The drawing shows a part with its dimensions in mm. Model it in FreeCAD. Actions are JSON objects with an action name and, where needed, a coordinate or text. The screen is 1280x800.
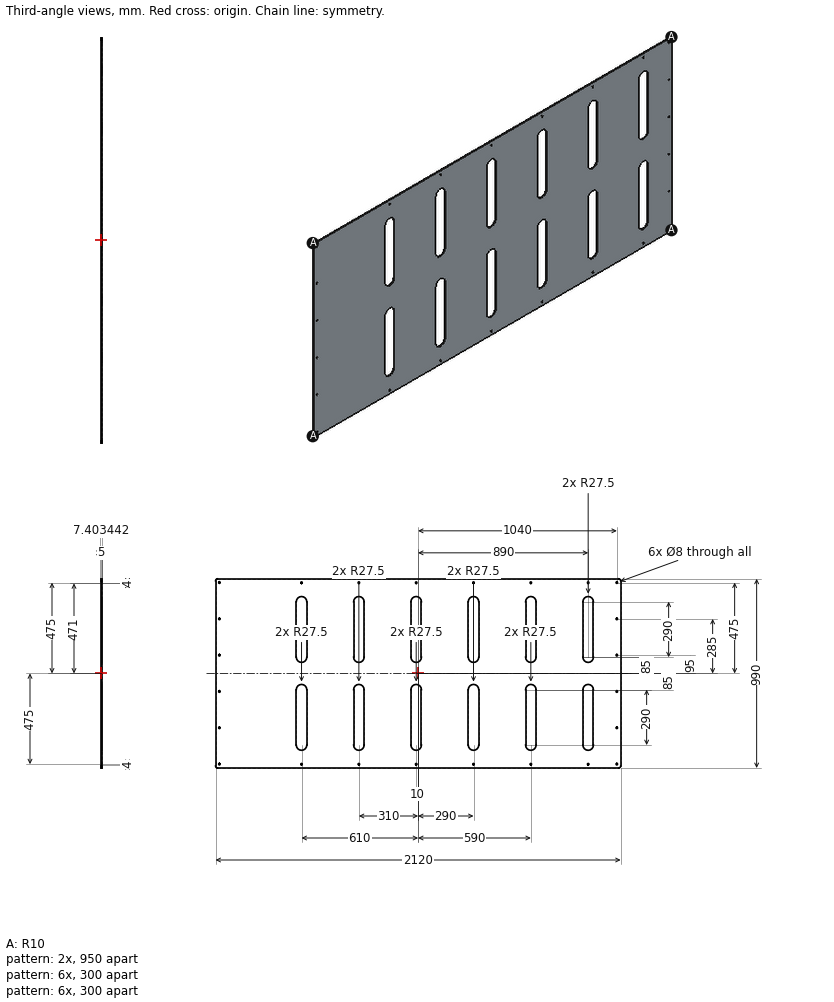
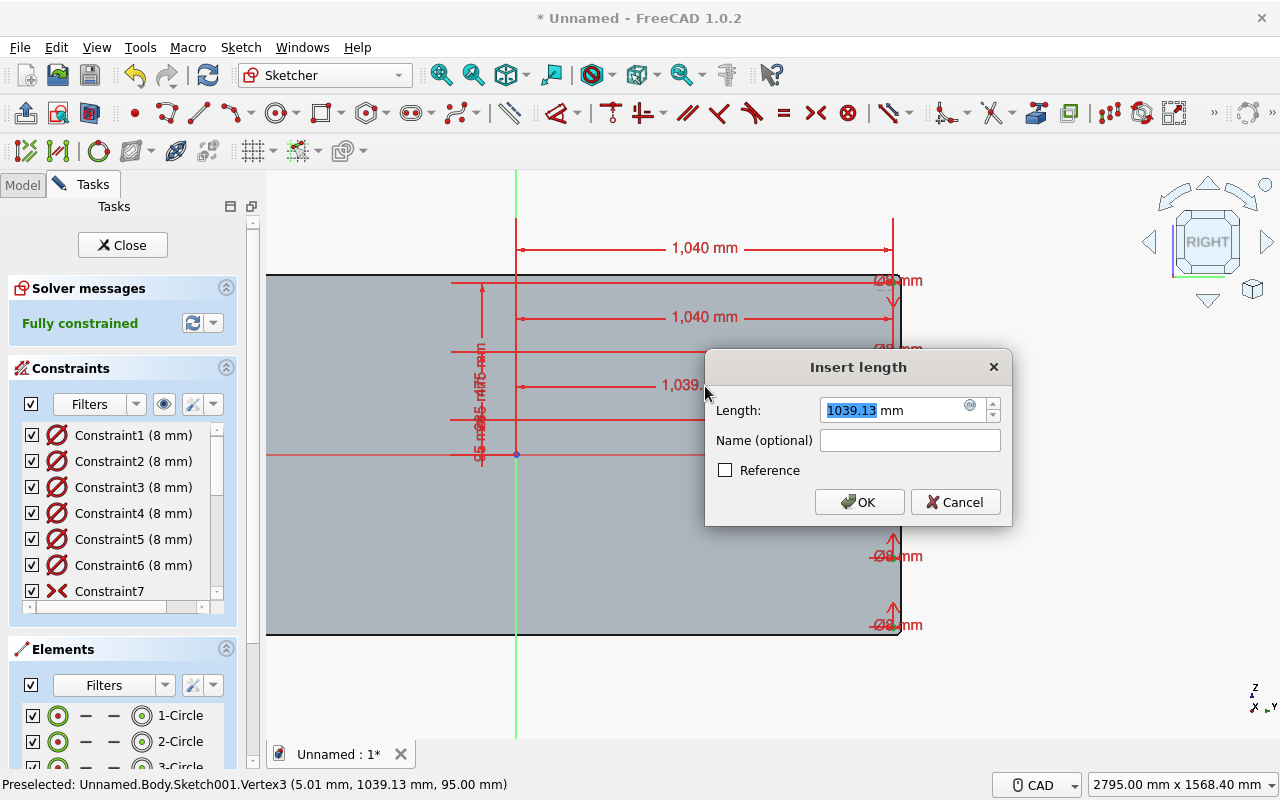
{"action": "type", "text": "1040"}
{"action": "key", "text": "Return"}
{"action": "key", "text": "Escape"}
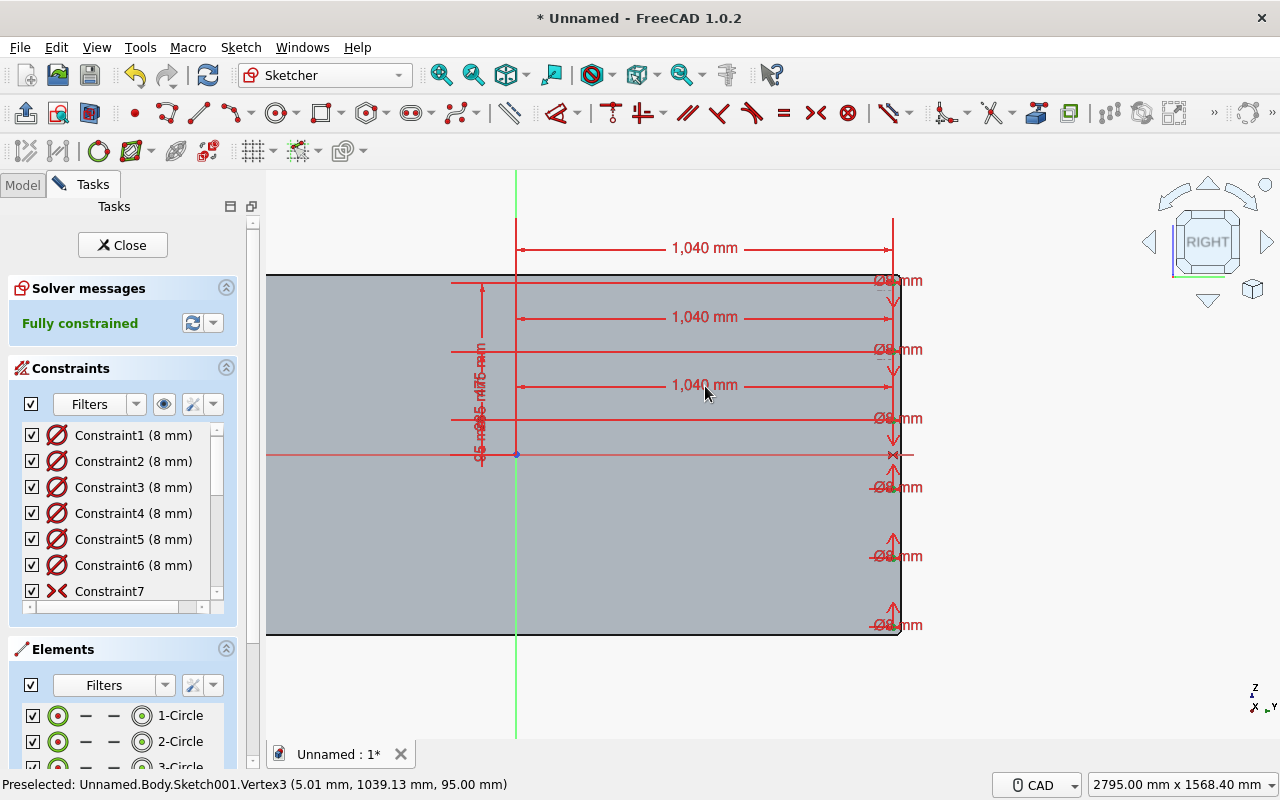
{"action": "left_click", "coordinate": [123, 245]}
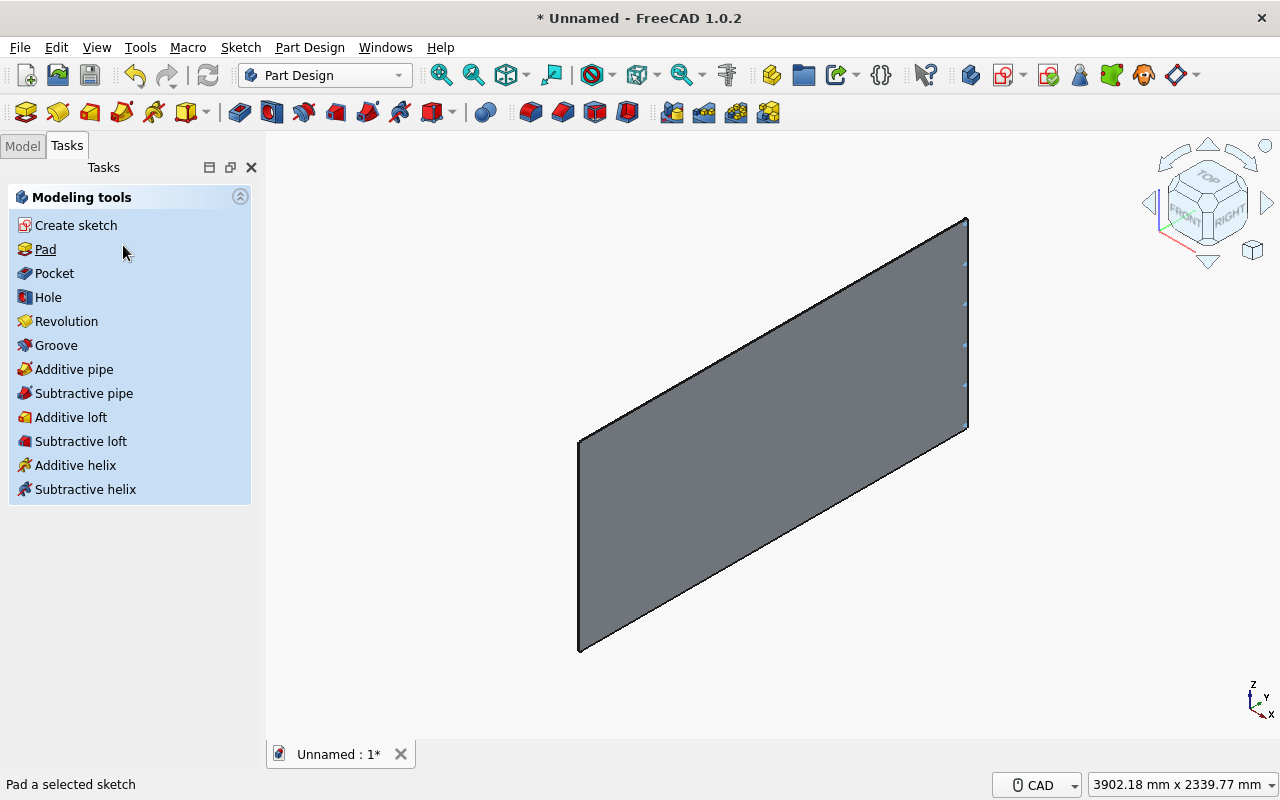
{"action": "left_click", "coordinate": [272, 112]}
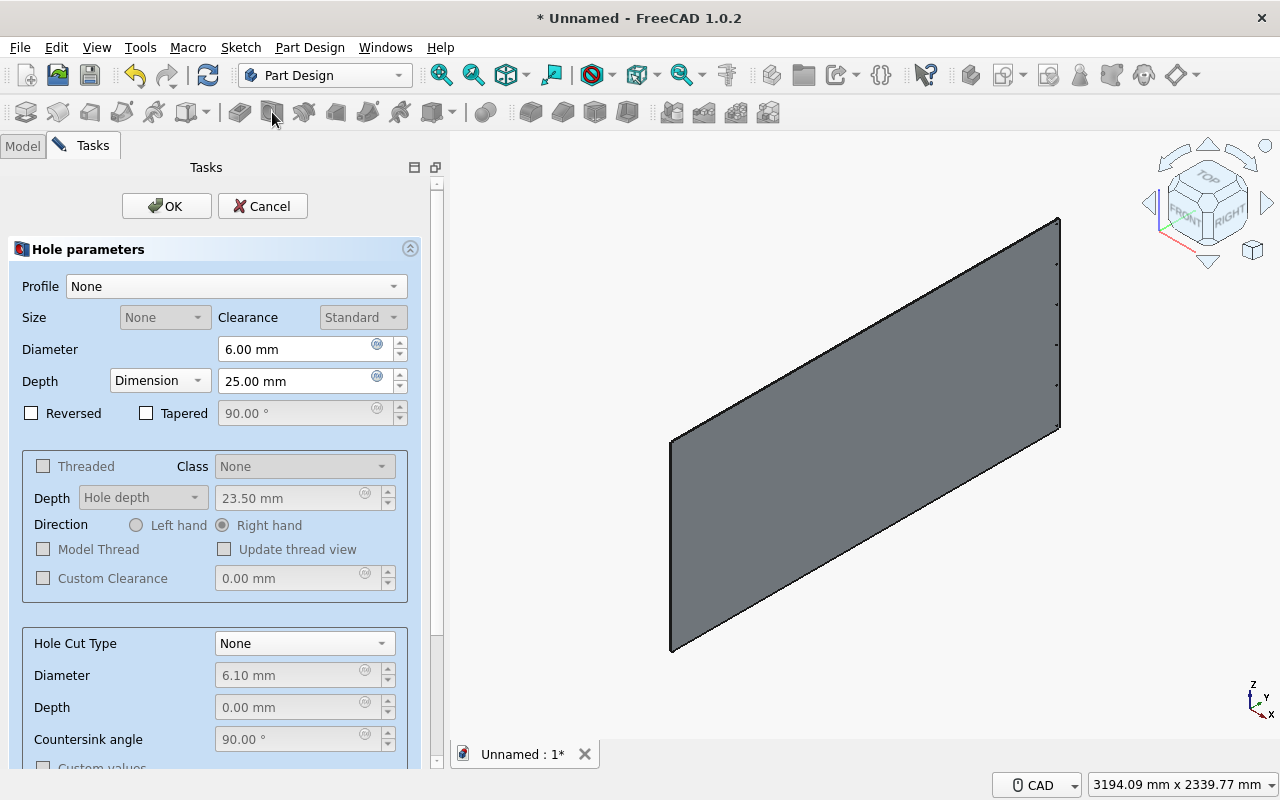
{"action": "triple_click", "coordinate": [305, 349]}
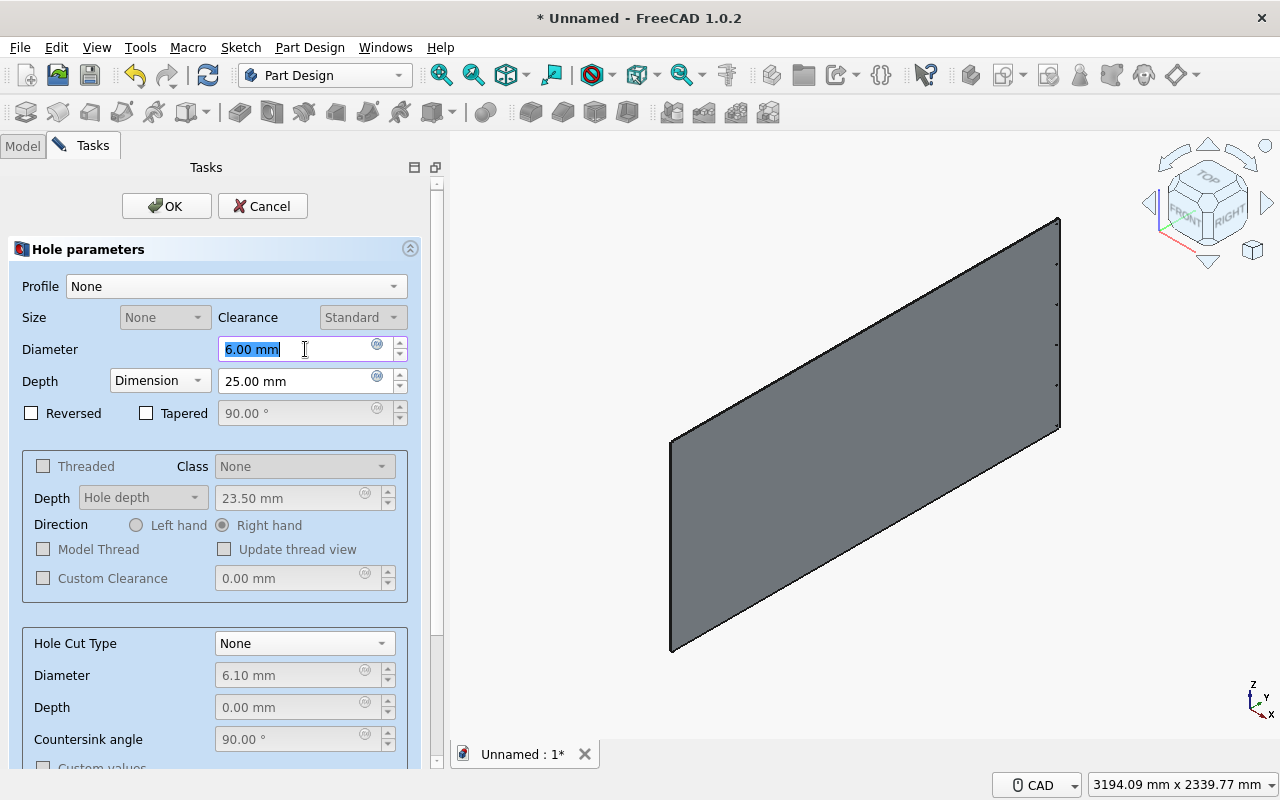
{"action": "type", "text": "8"}
{"action": "key", "text": "Tab"}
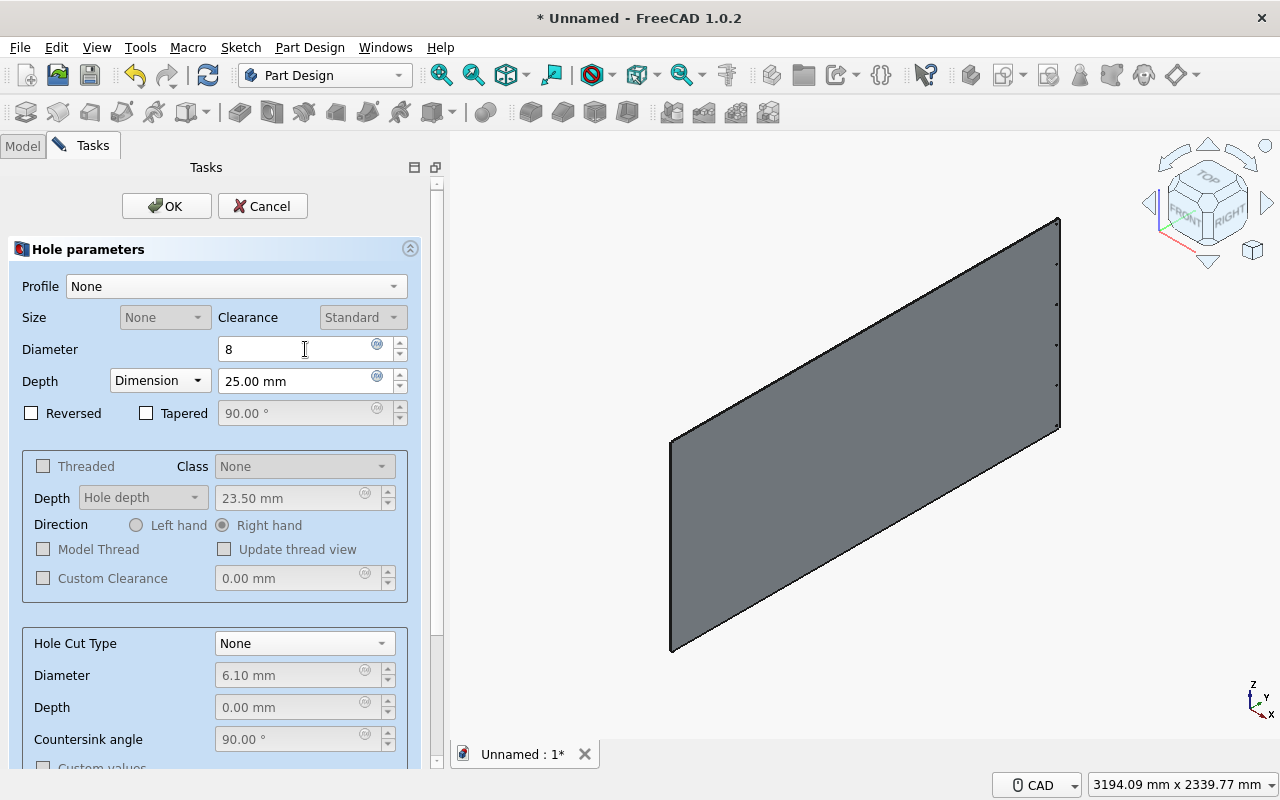
{"action": "left_click", "coordinate": [161, 380]}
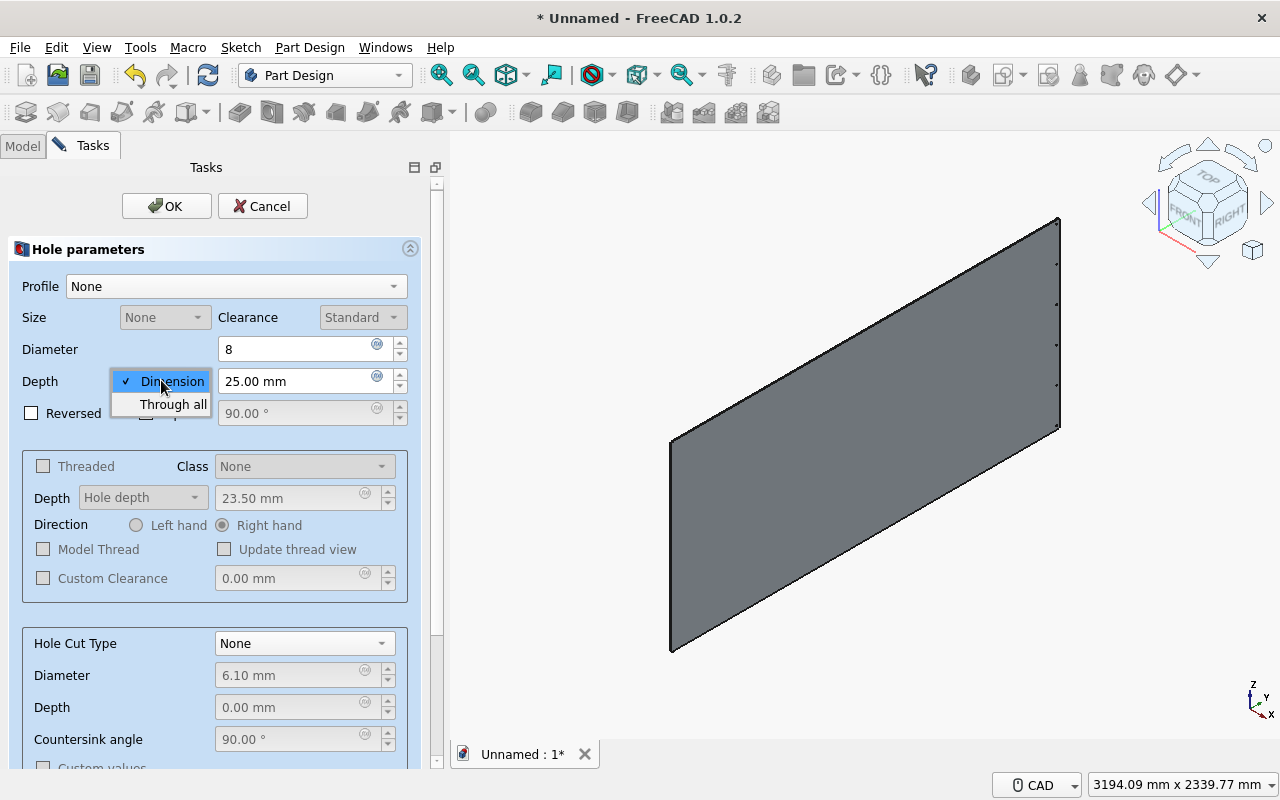
{"action": "left_click", "coordinate": [160, 404]}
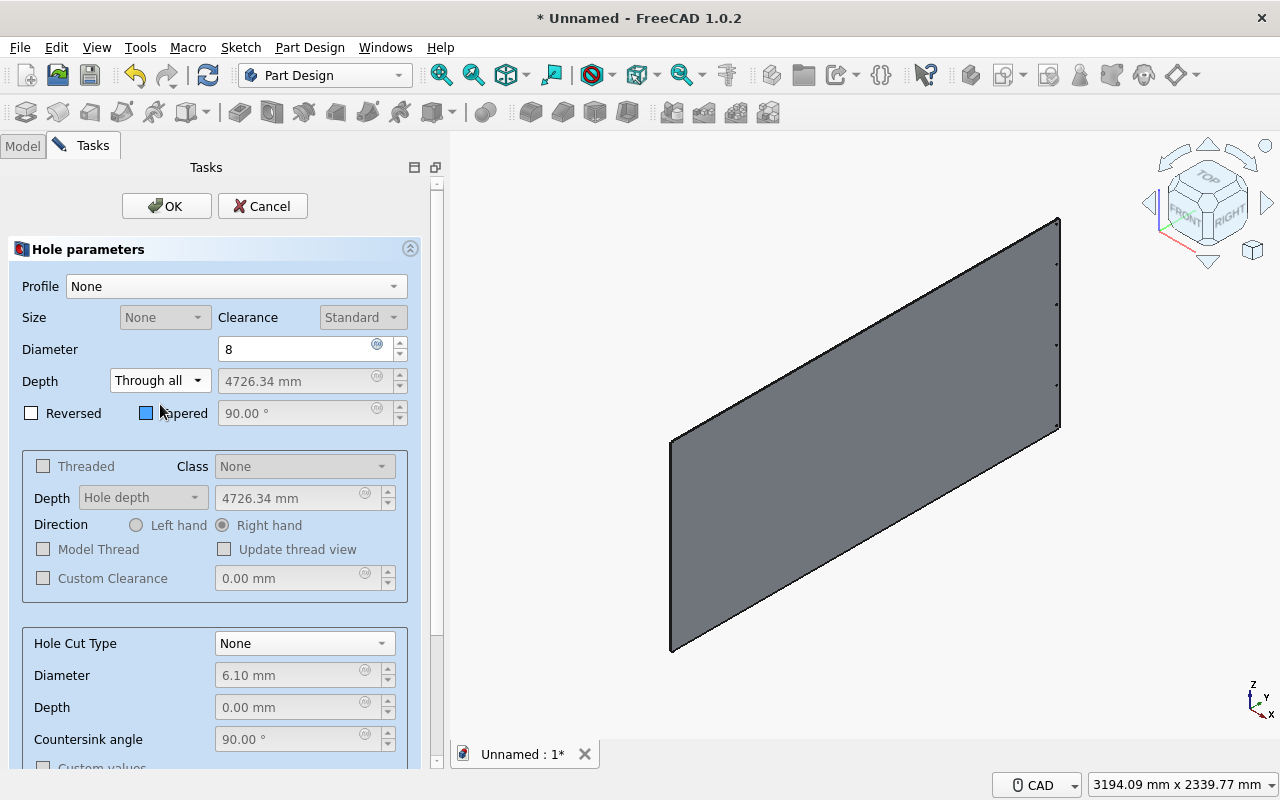
{"action": "left_click", "coordinate": [167, 206]}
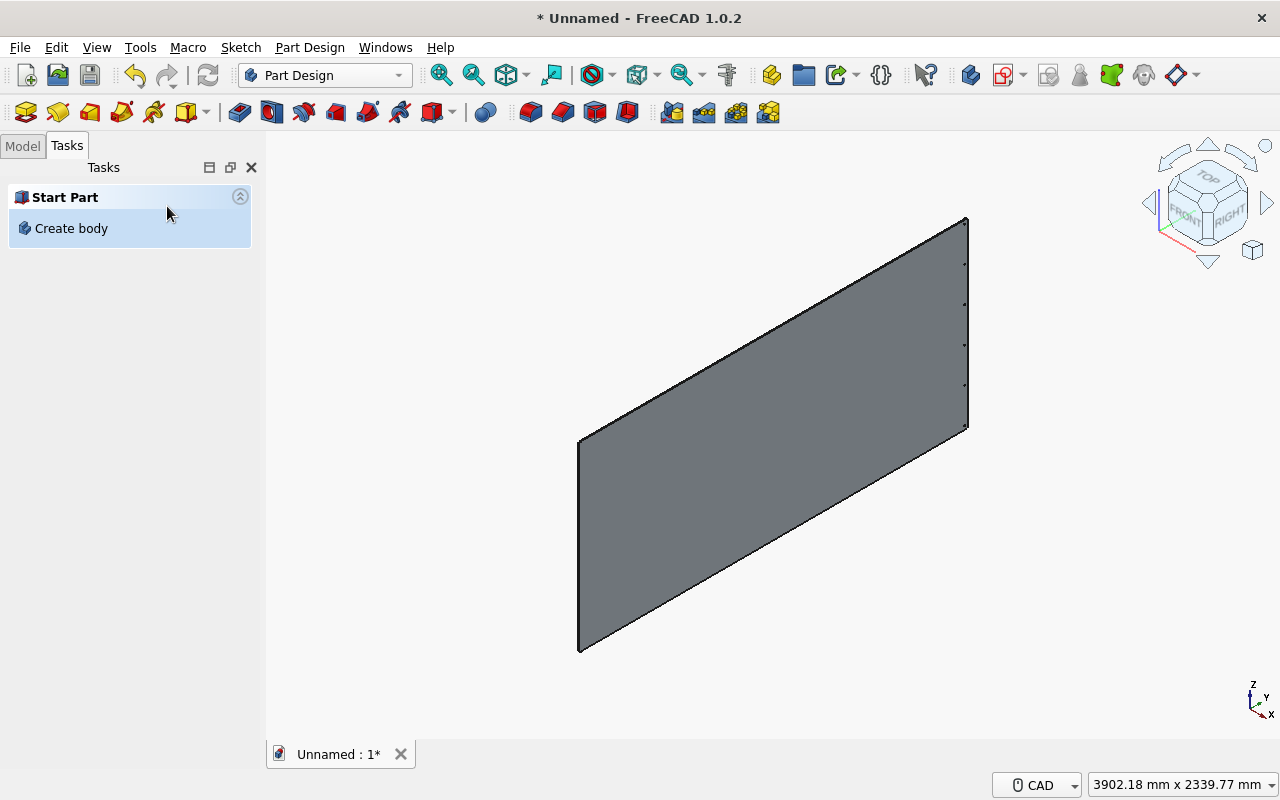
{"action": "left_click", "coordinate": [23, 145]}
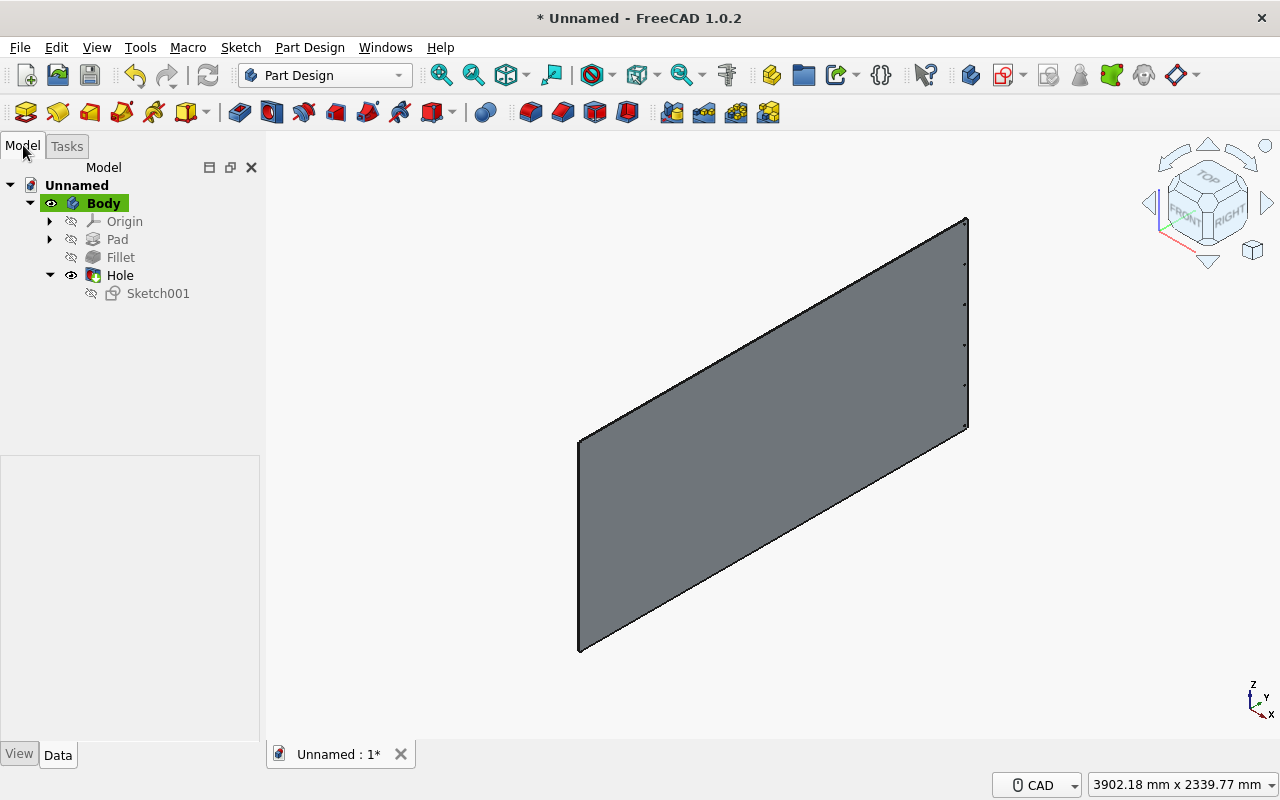
{"action": "left_click", "coordinate": [116, 275]}